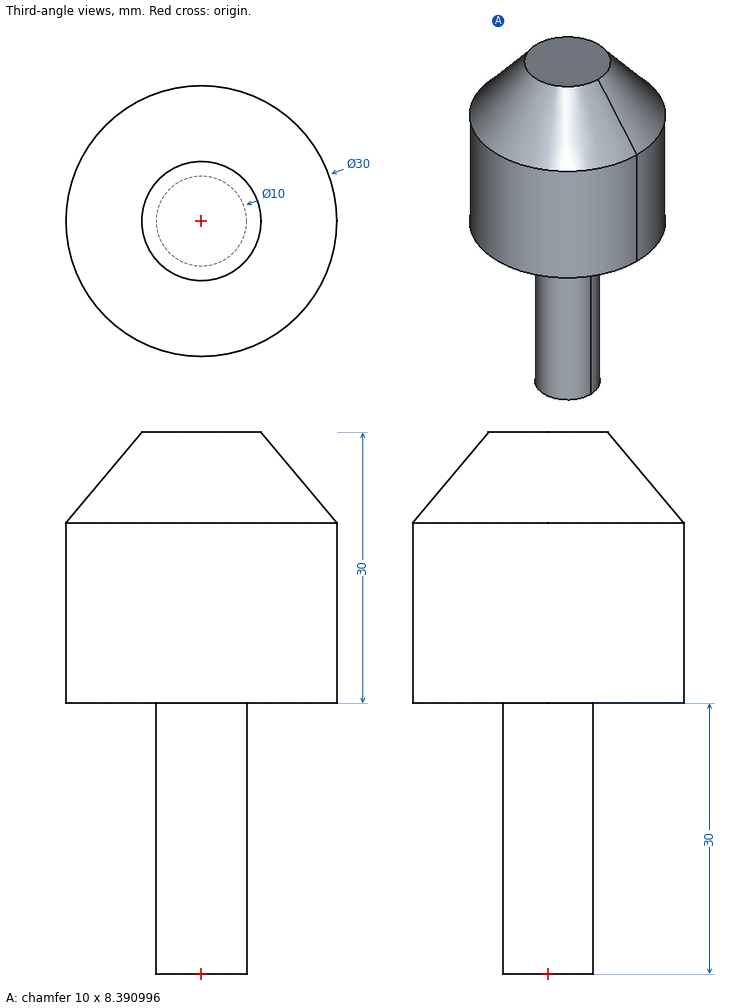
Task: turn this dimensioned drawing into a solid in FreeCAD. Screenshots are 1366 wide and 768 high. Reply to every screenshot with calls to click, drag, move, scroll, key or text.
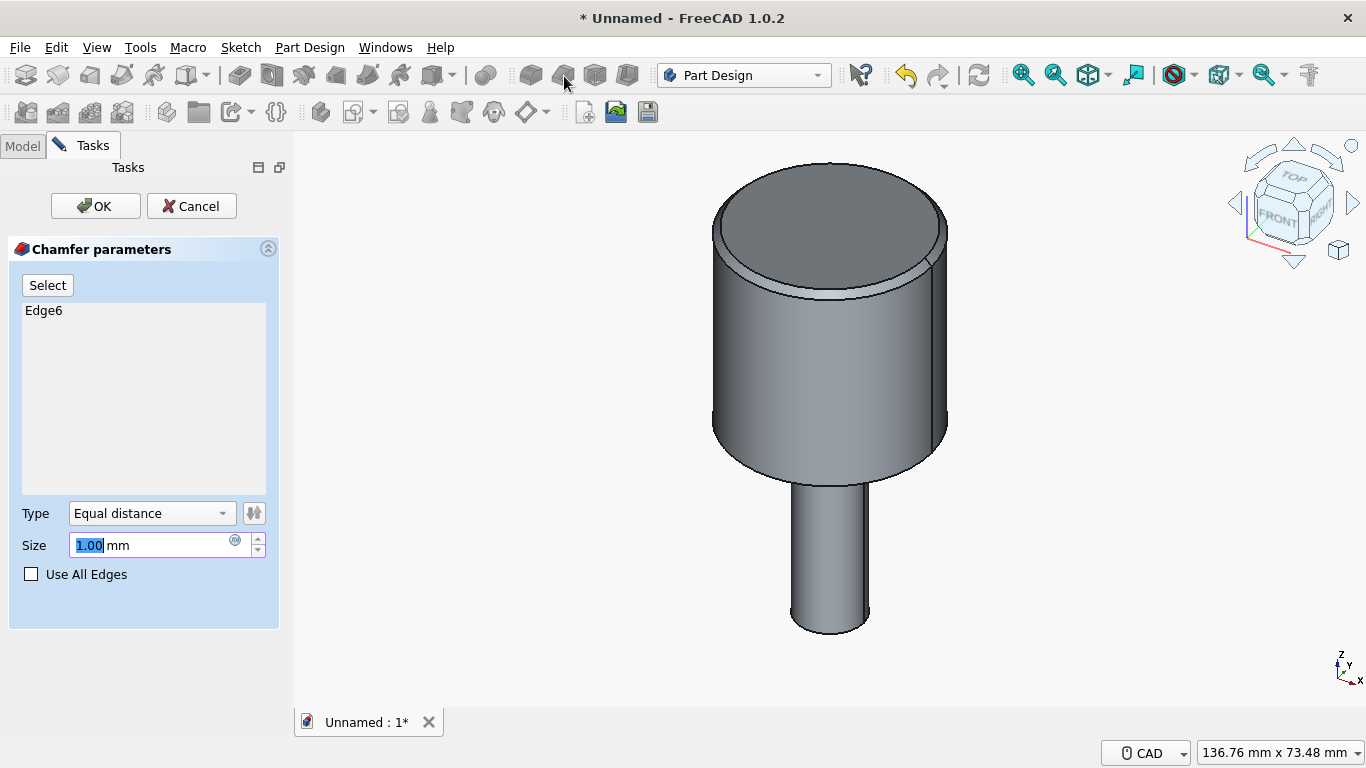
text(10)
key(Tab)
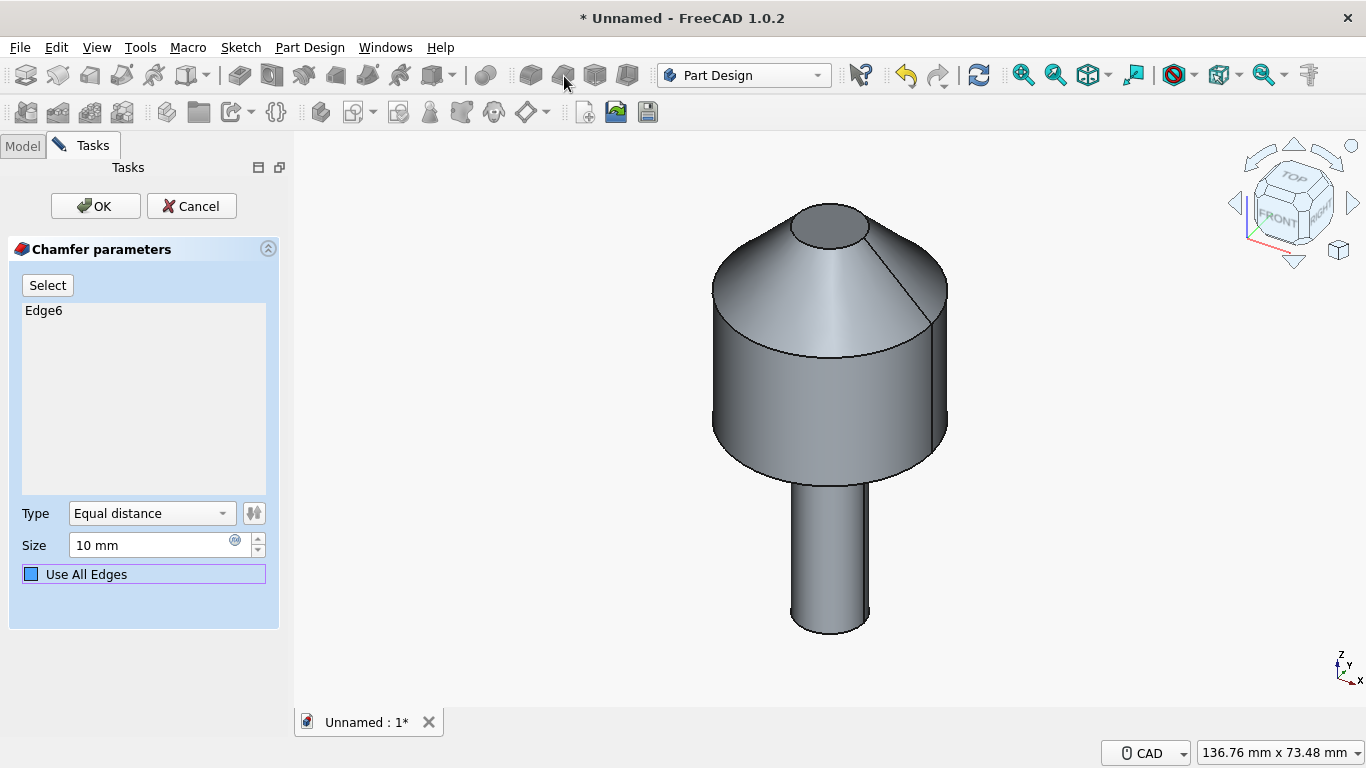
click(153, 514)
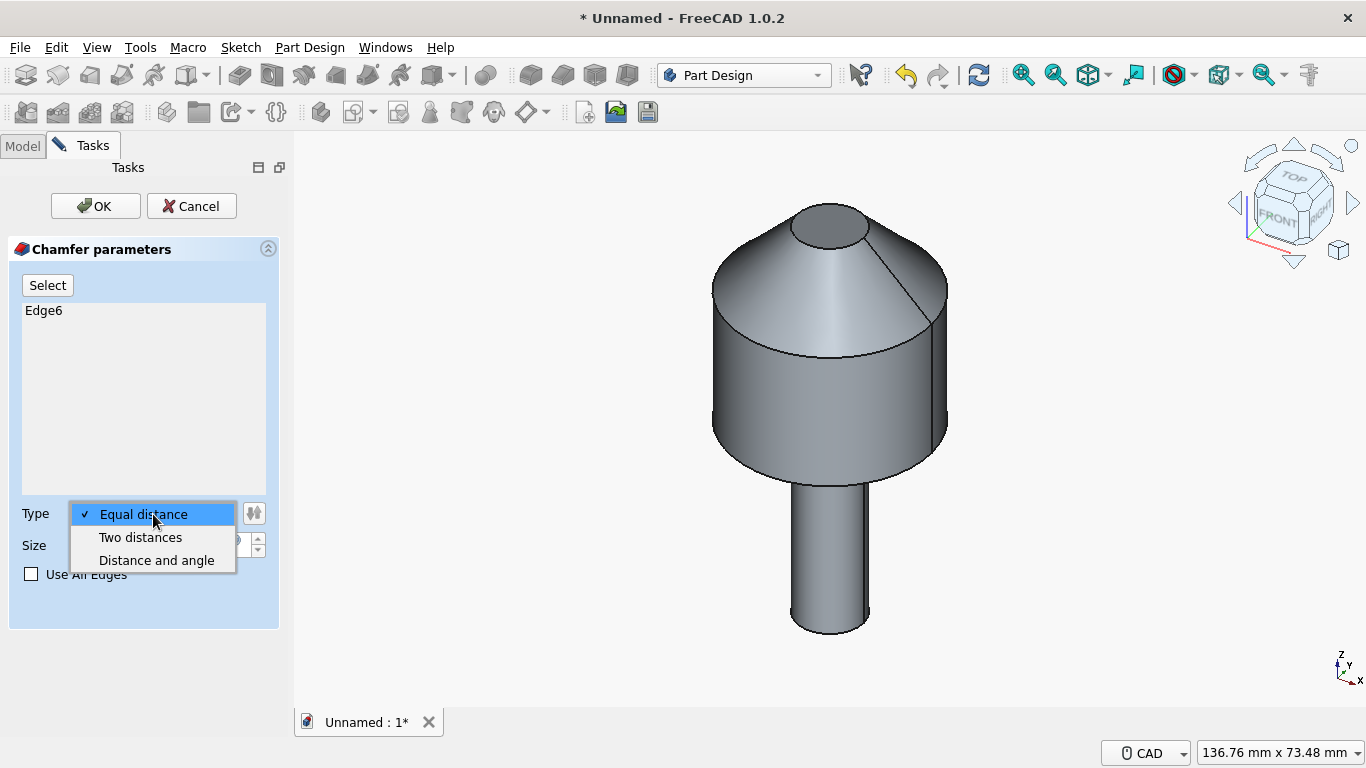
click(152, 538)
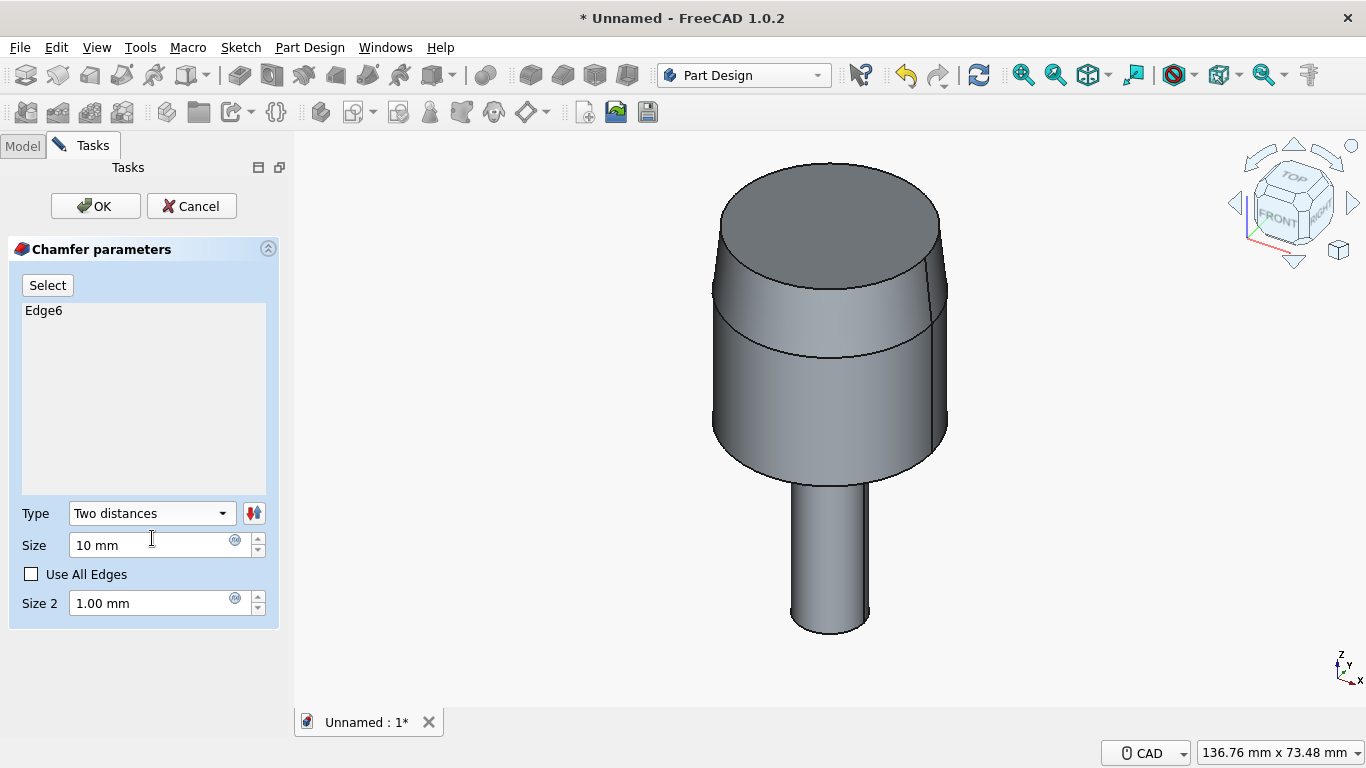
triple_click(160, 603)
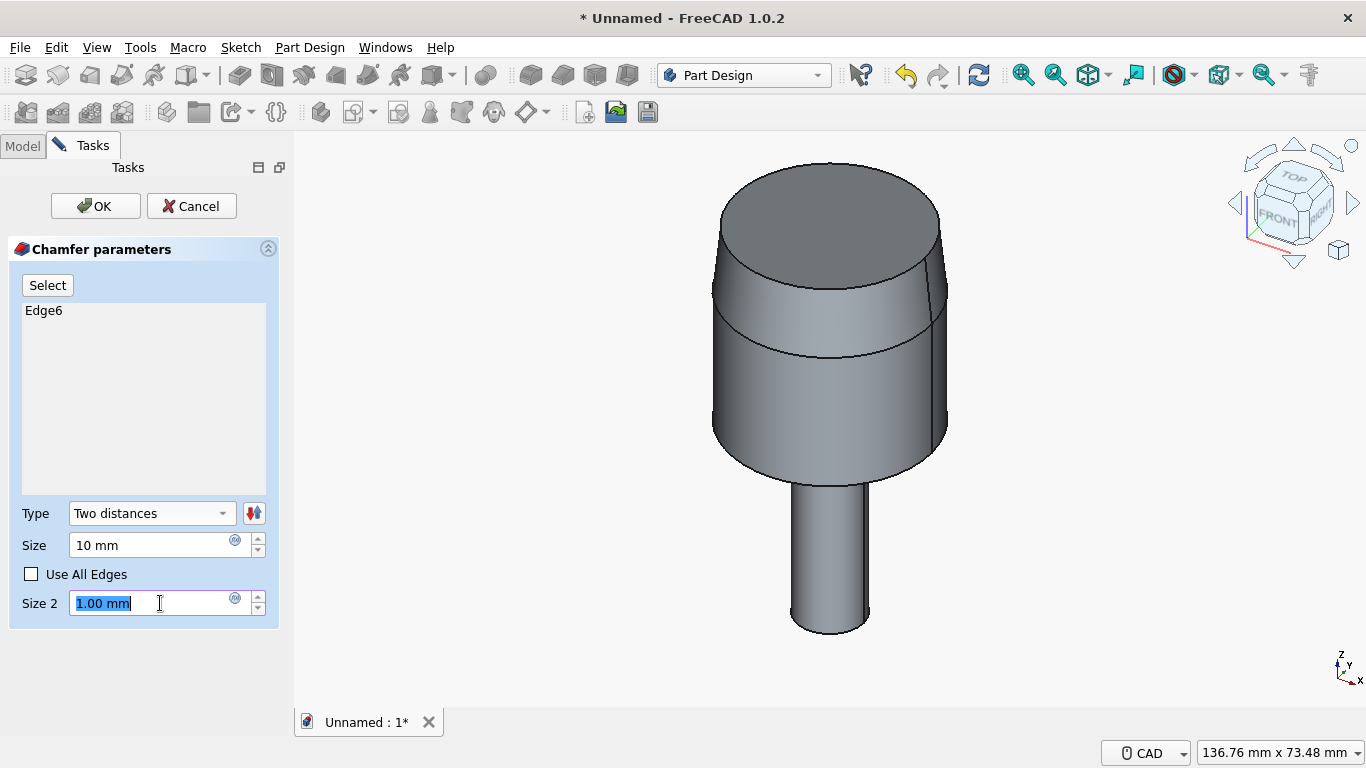
text(8.390996)
key(Tab)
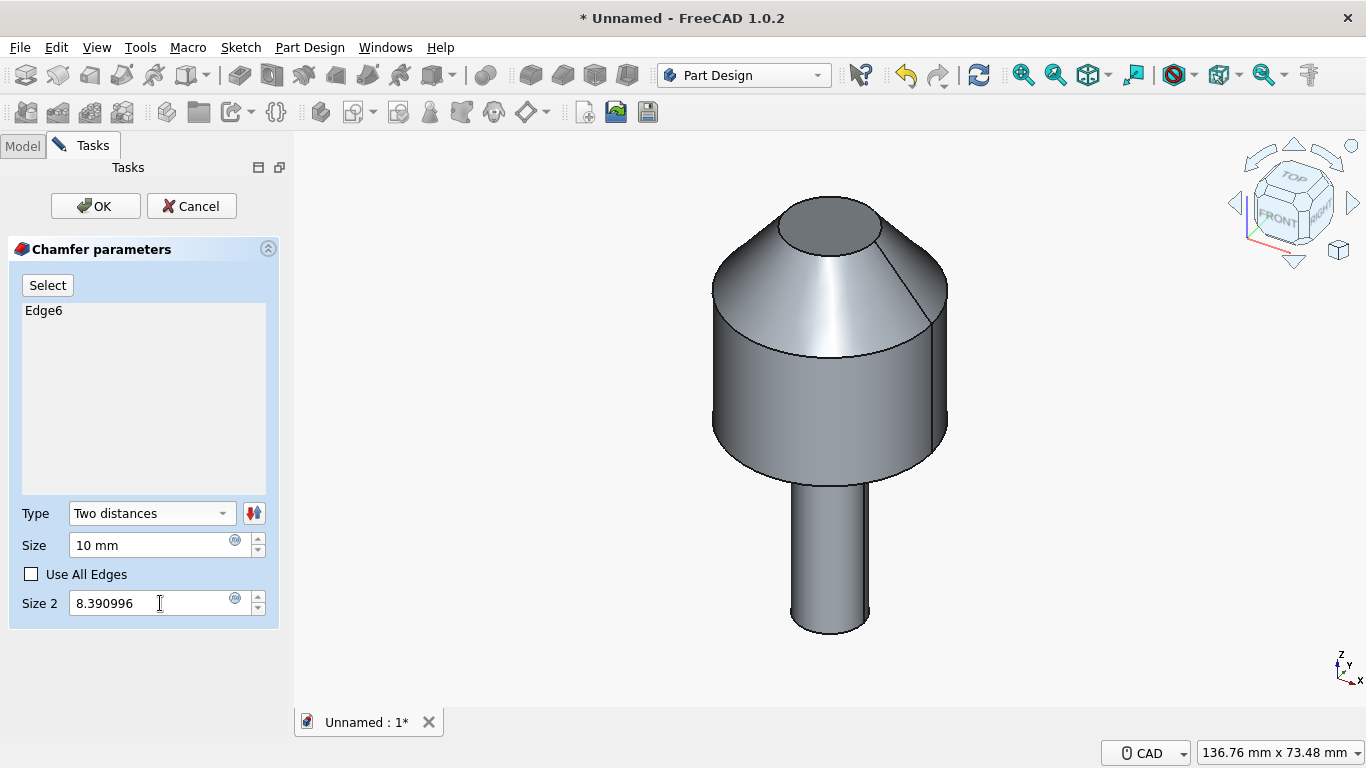
click(96, 206)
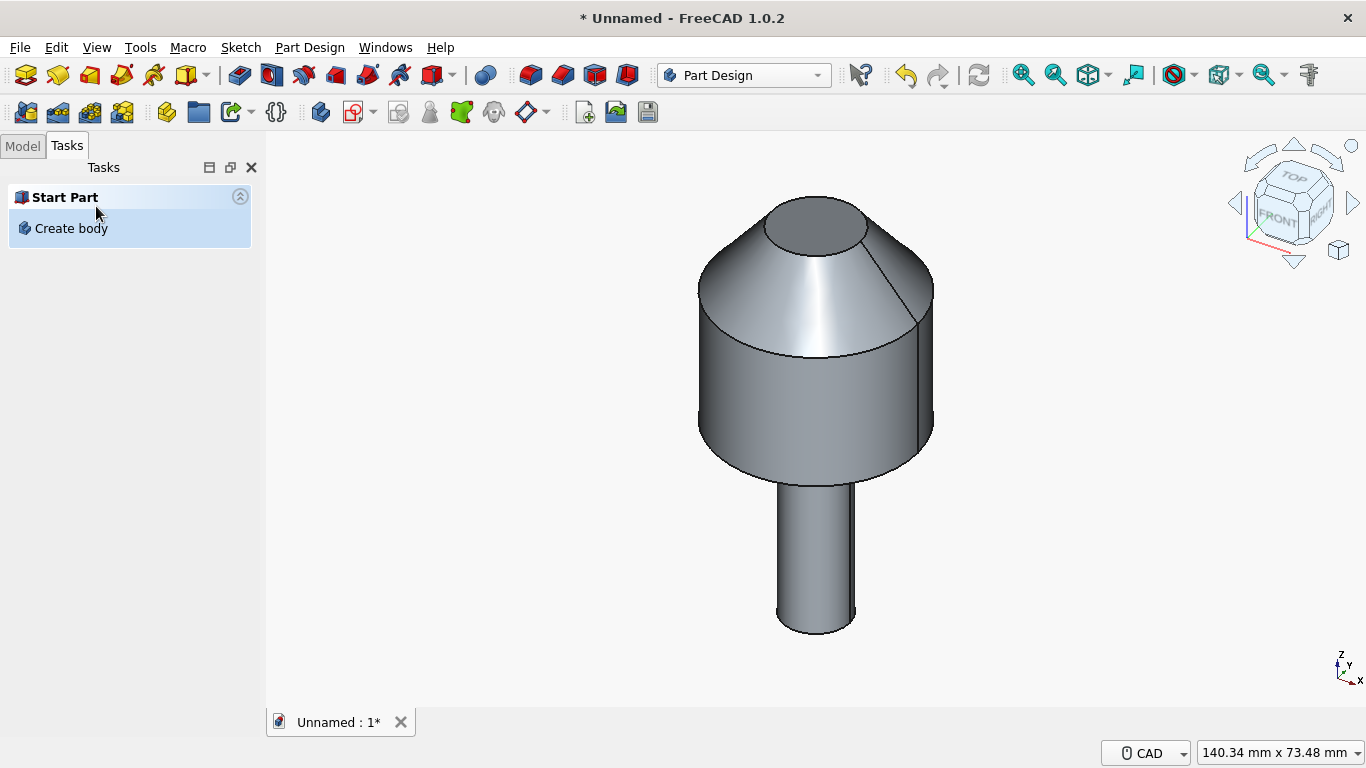
key(0)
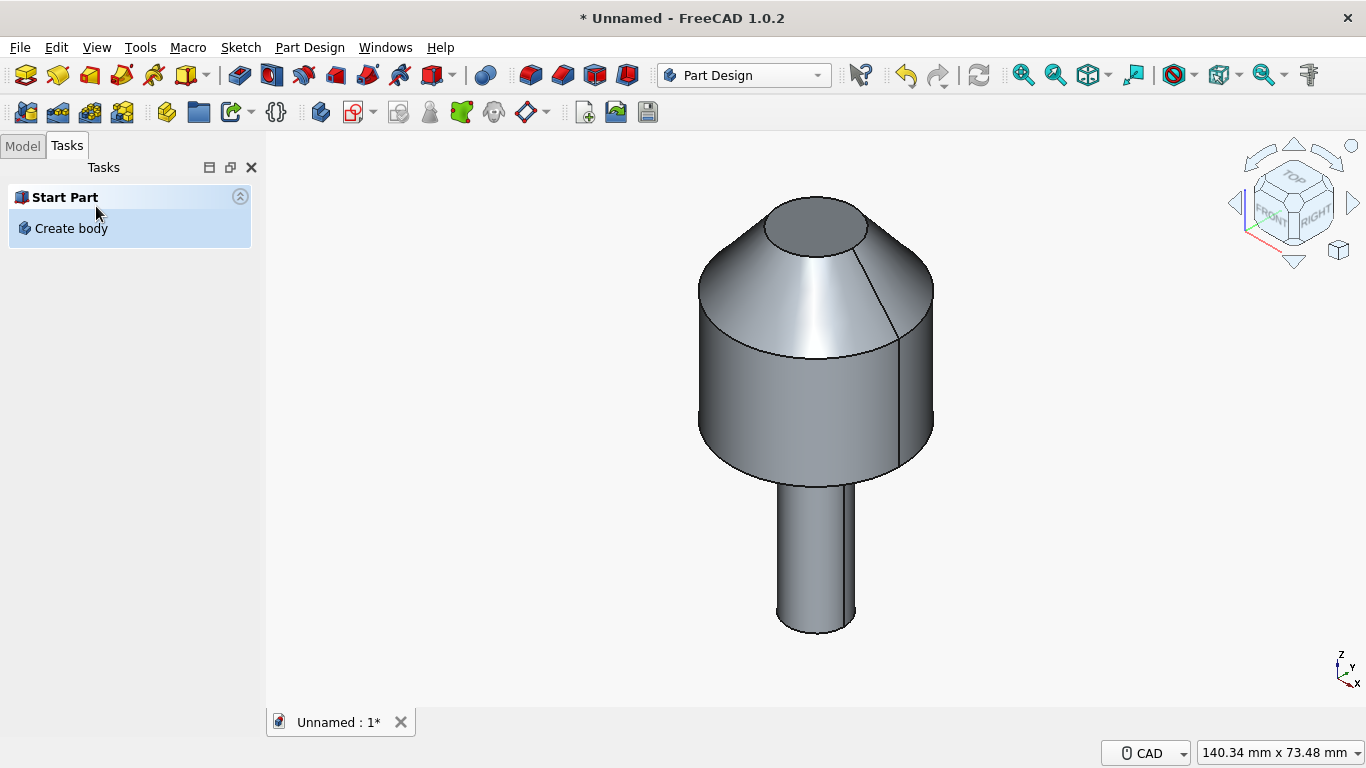
click(1024, 76)